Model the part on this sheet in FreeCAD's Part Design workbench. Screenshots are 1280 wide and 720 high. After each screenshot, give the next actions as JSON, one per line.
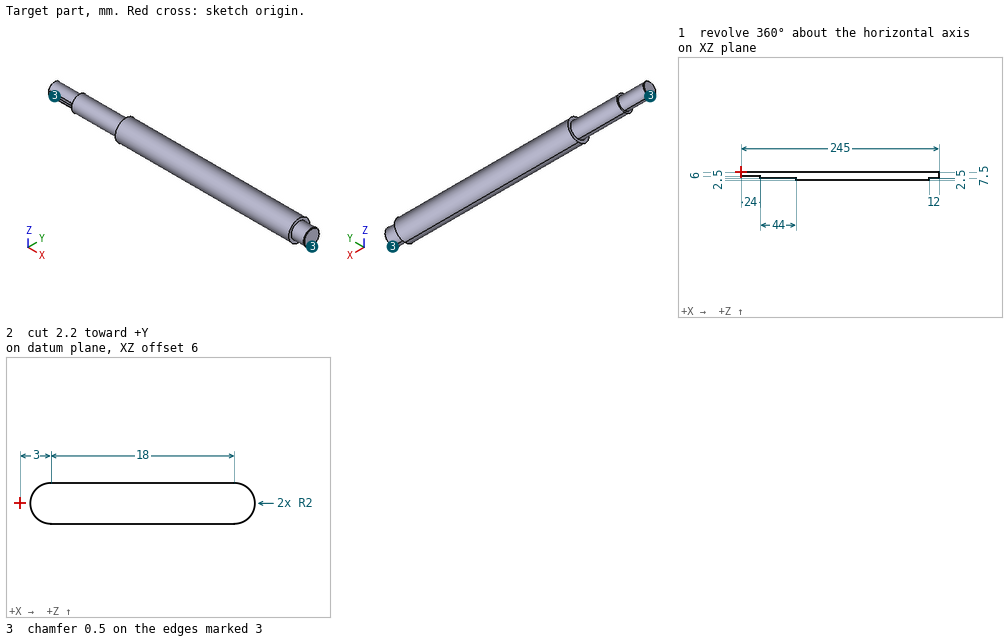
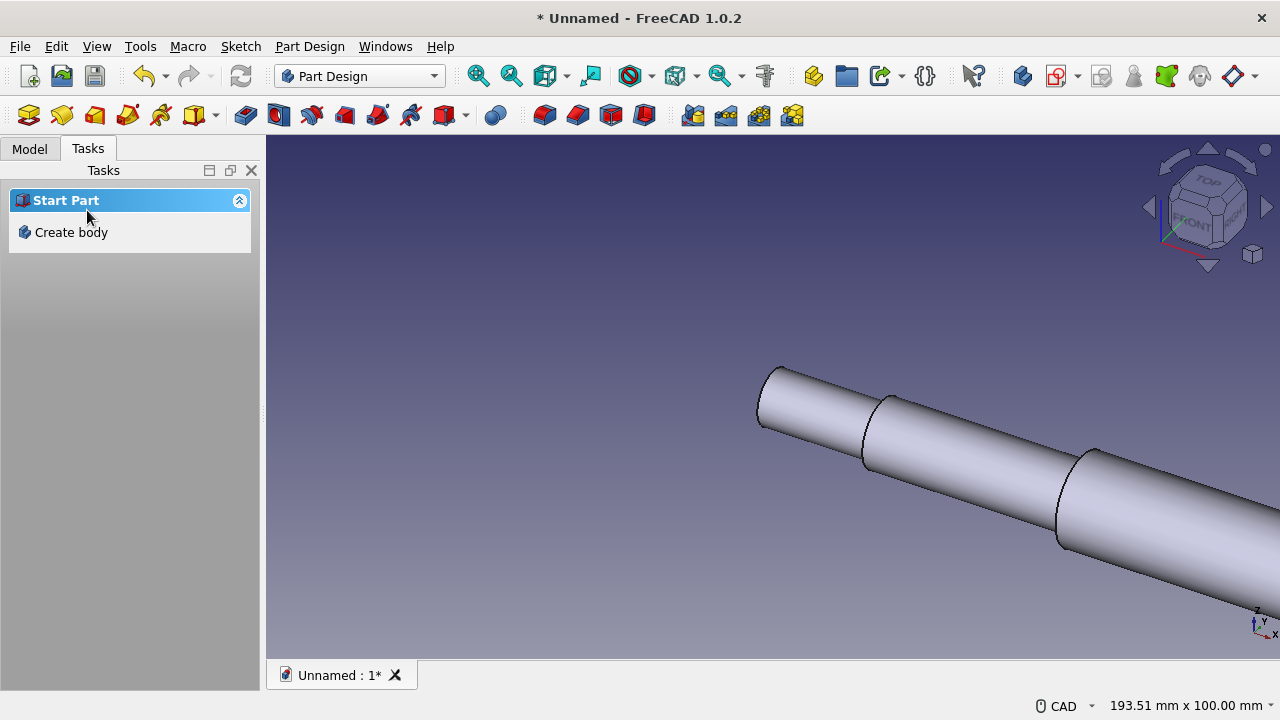
{"action": "left_click", "coordinate": [479, 76]}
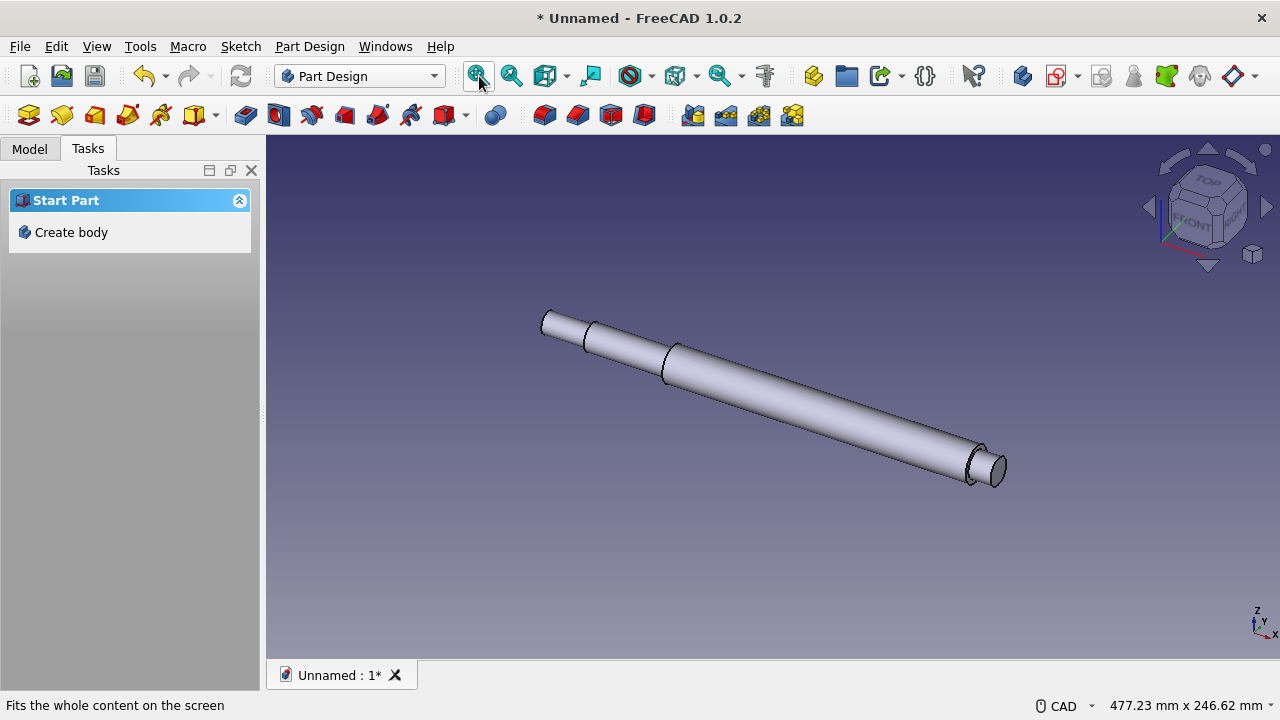
{"action": "left_click", "coordinate": [30, 148]}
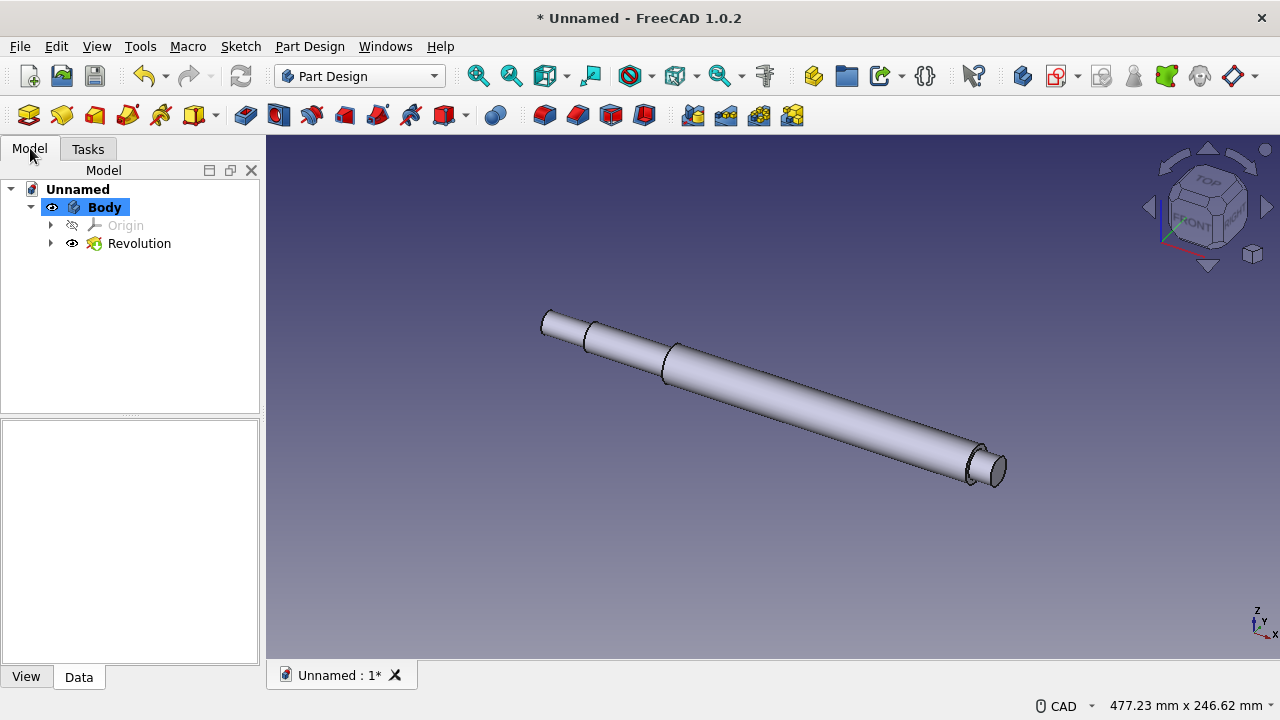
{"action": "left_click", "coordinate": [51, 225]}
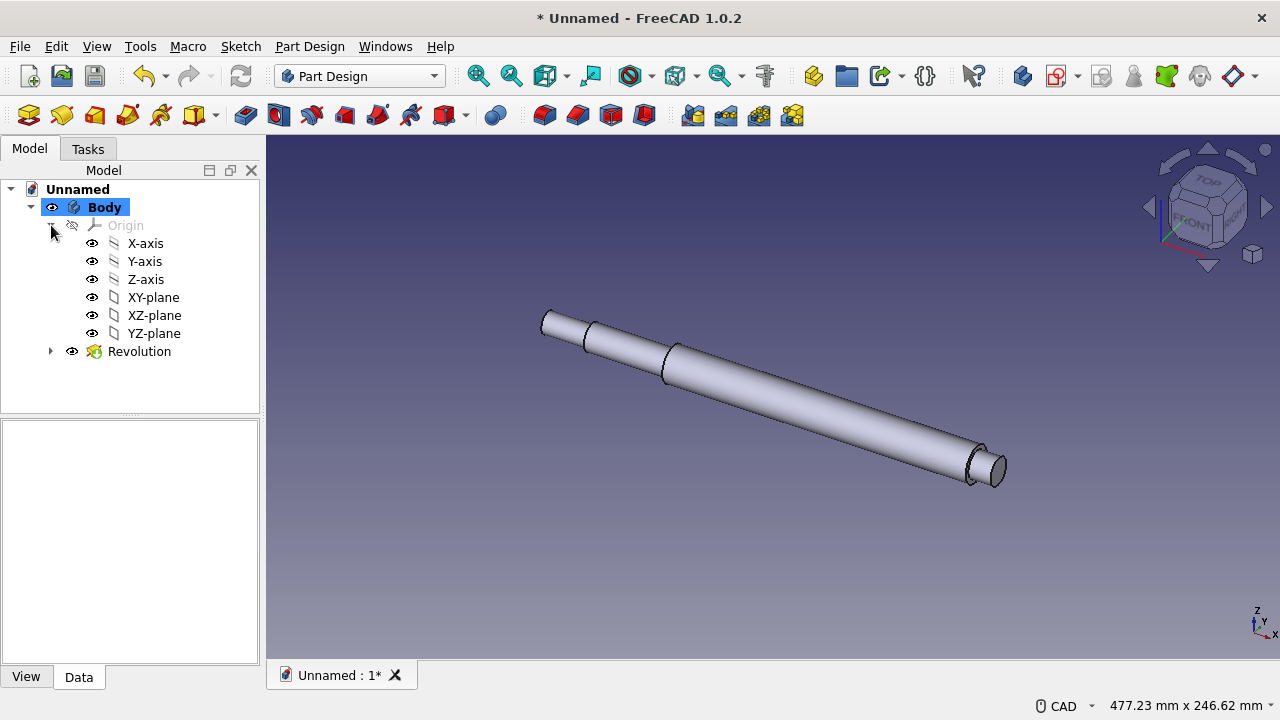
{"action": "left_click", "coordinate": [137, 315]}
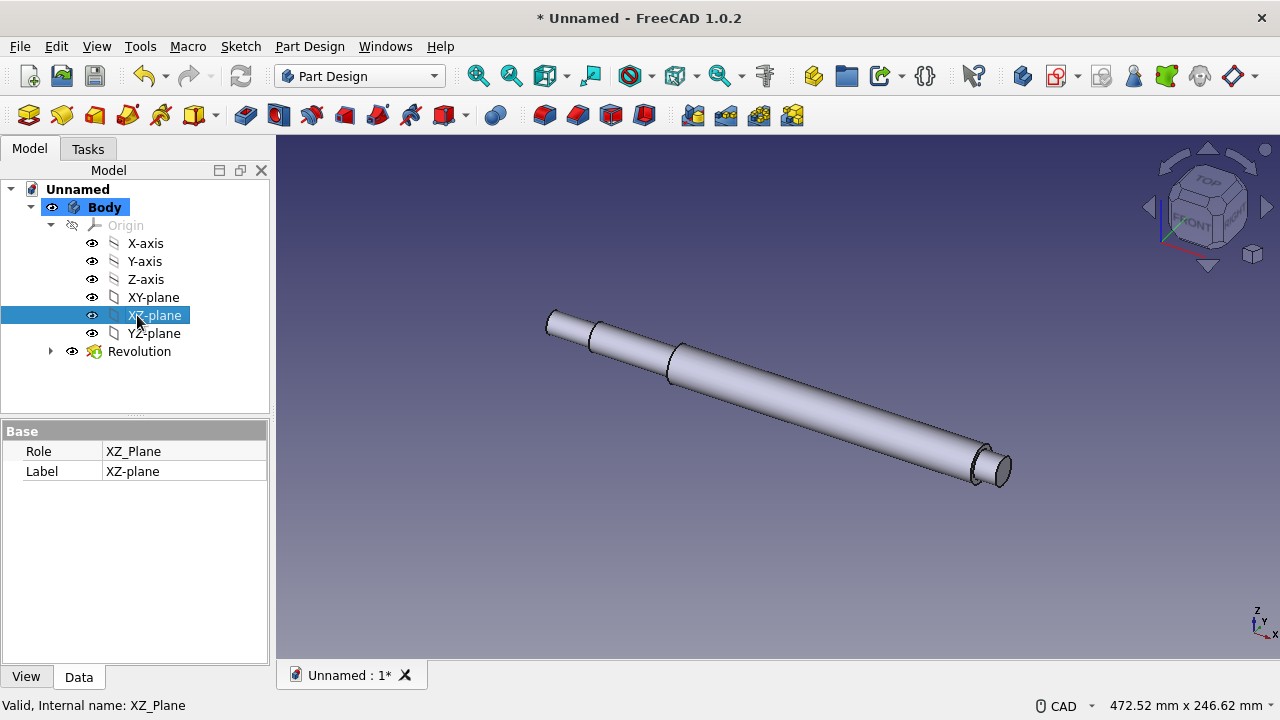
{"action": "left_click", "coordinate": [1232, 76]}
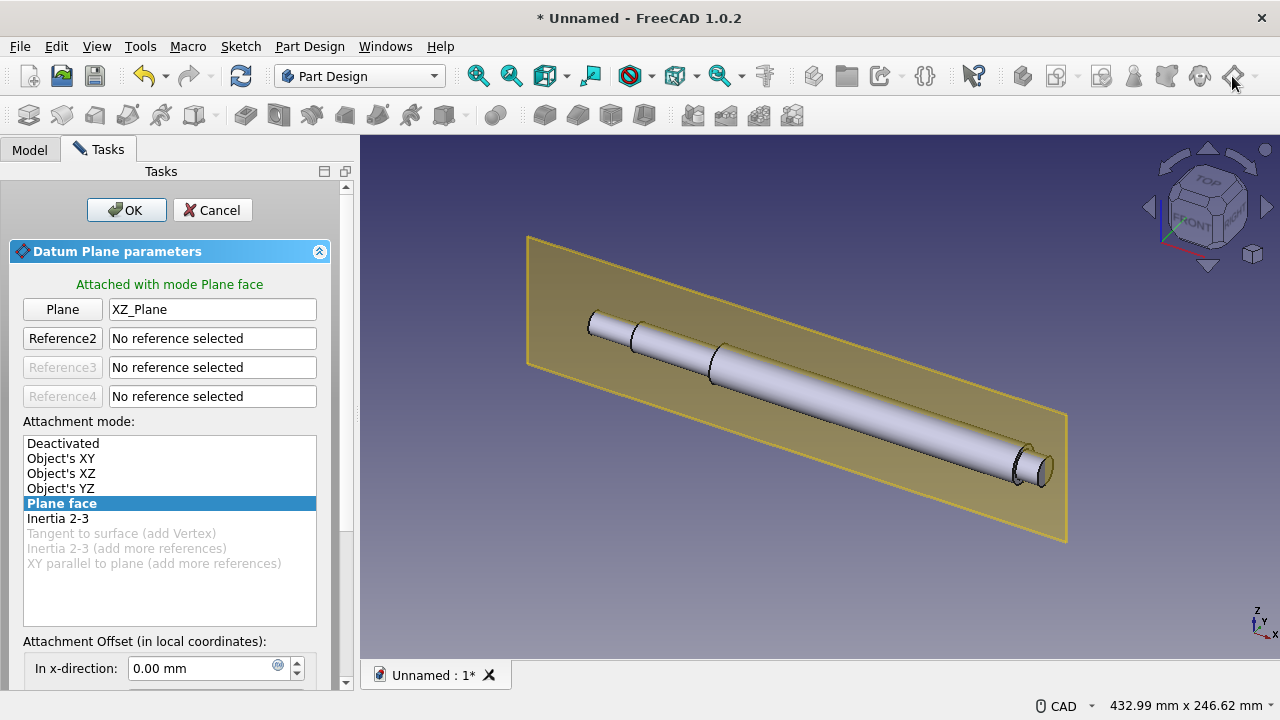
{"action": "scroll", "coordinate": [346, 436], "scroll_direction": "down", "scroll_amount": 2}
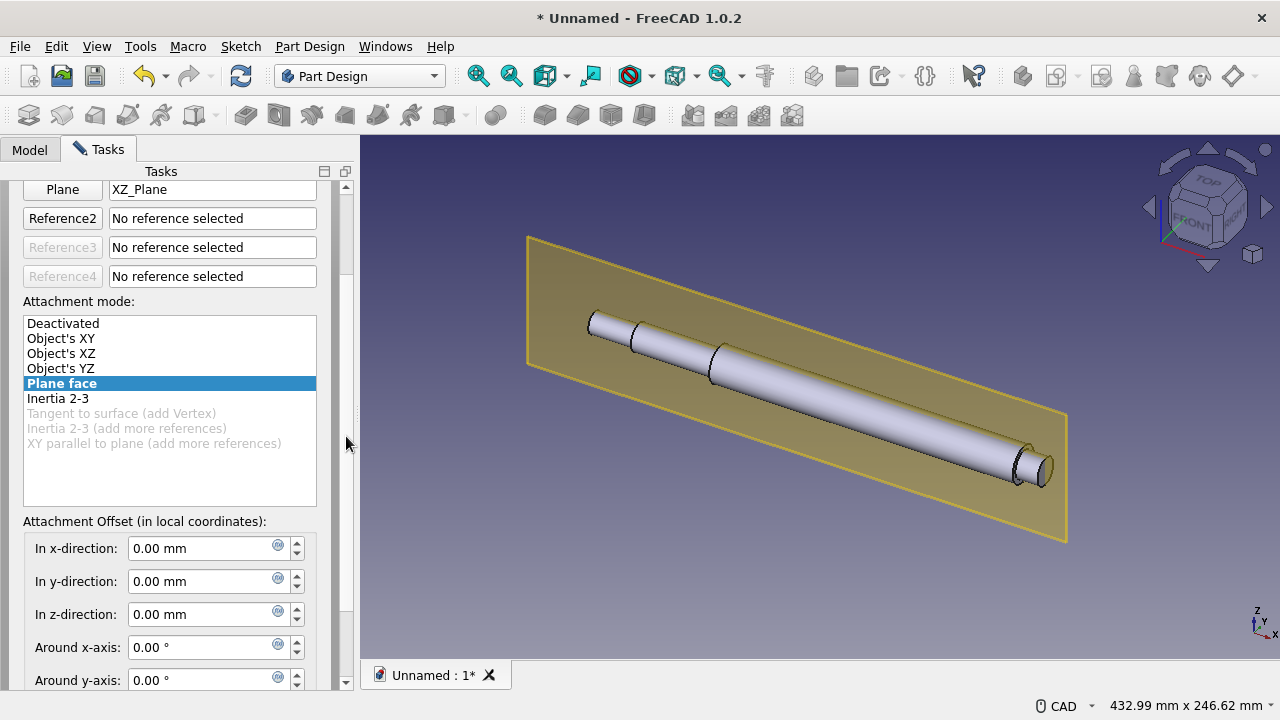
{"action": "triple_click", "coordinate": [210, 614]}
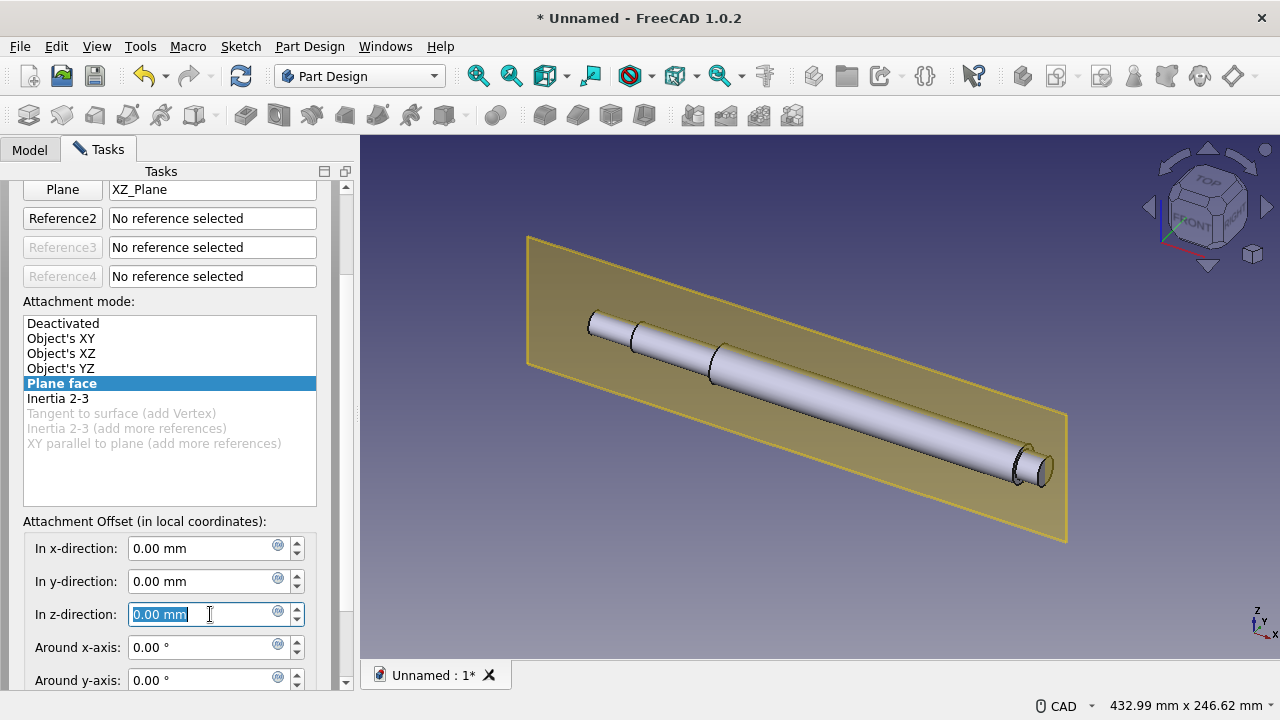
{"action": "type", "text": "6"}
{"action": "key", "text": "Tab"}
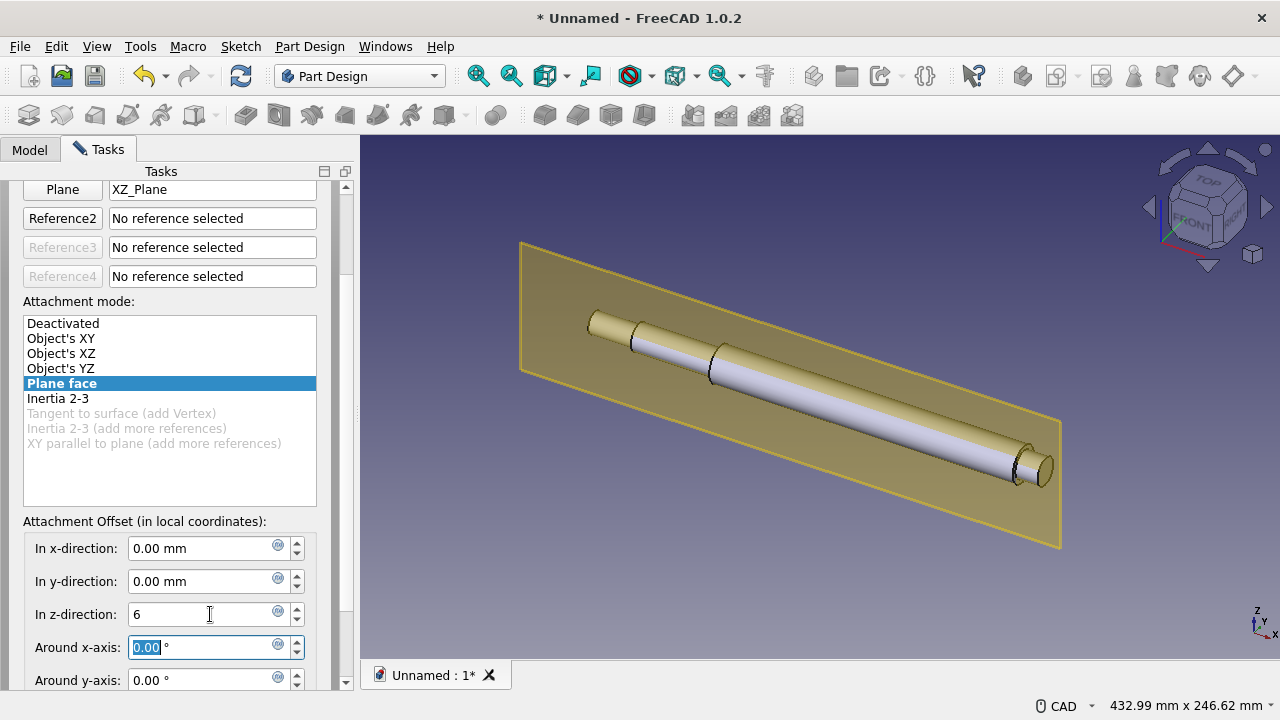
{"action": "scroll", "coordinate": [346, 436], "scroll_direction": "up", "scroll_amount": 3}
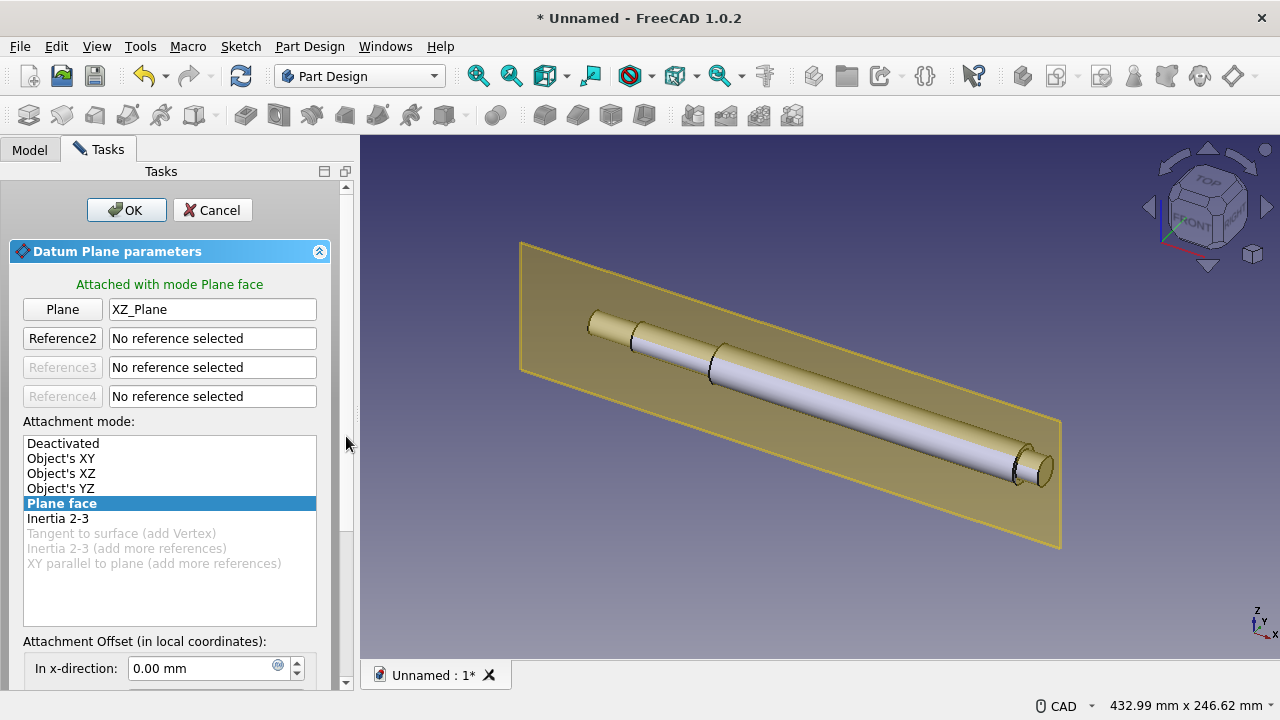
{"action": "left_click", "coordinate": [127, 210]}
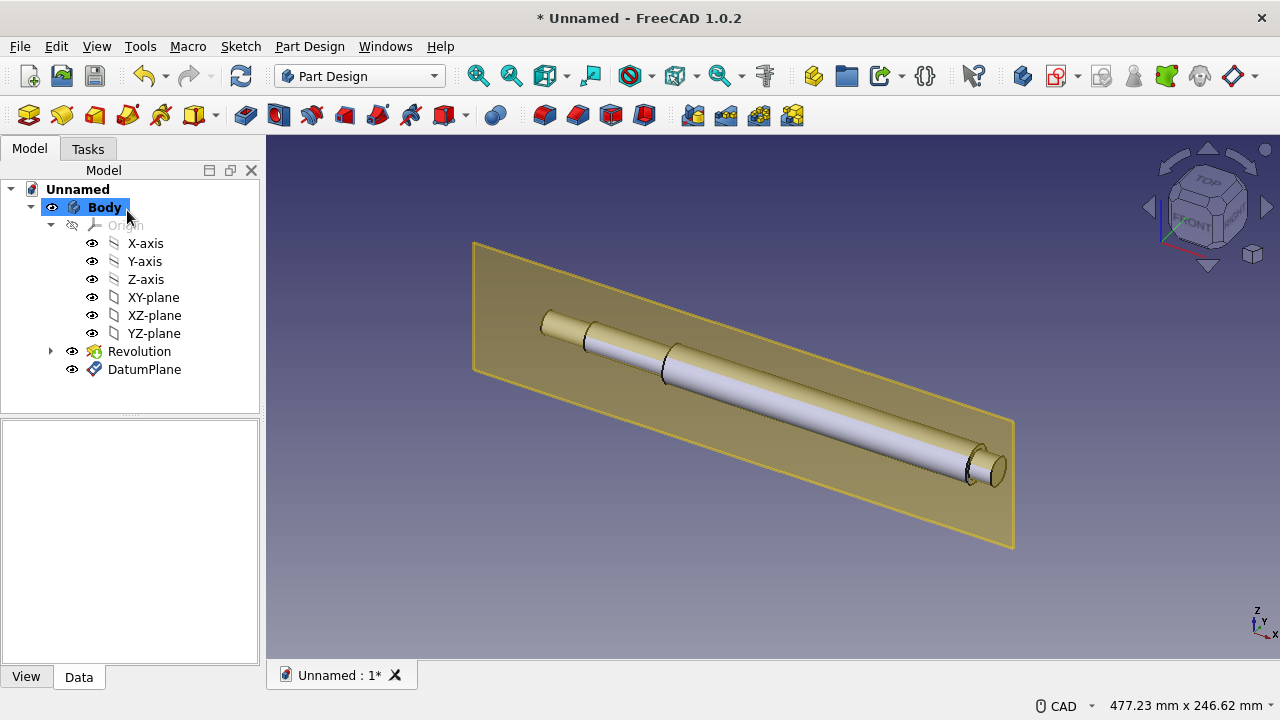
{"action": "left_click", "coordinate": [117, 369]}